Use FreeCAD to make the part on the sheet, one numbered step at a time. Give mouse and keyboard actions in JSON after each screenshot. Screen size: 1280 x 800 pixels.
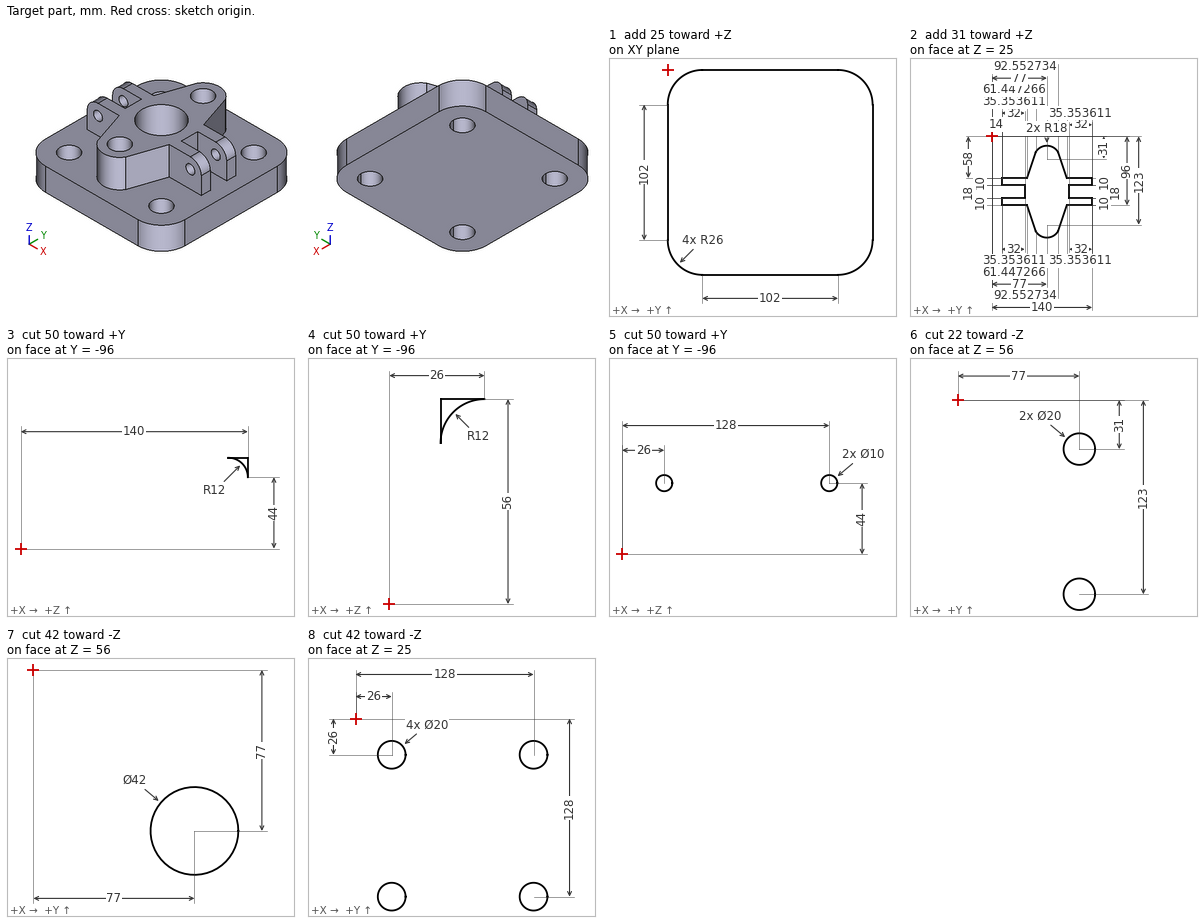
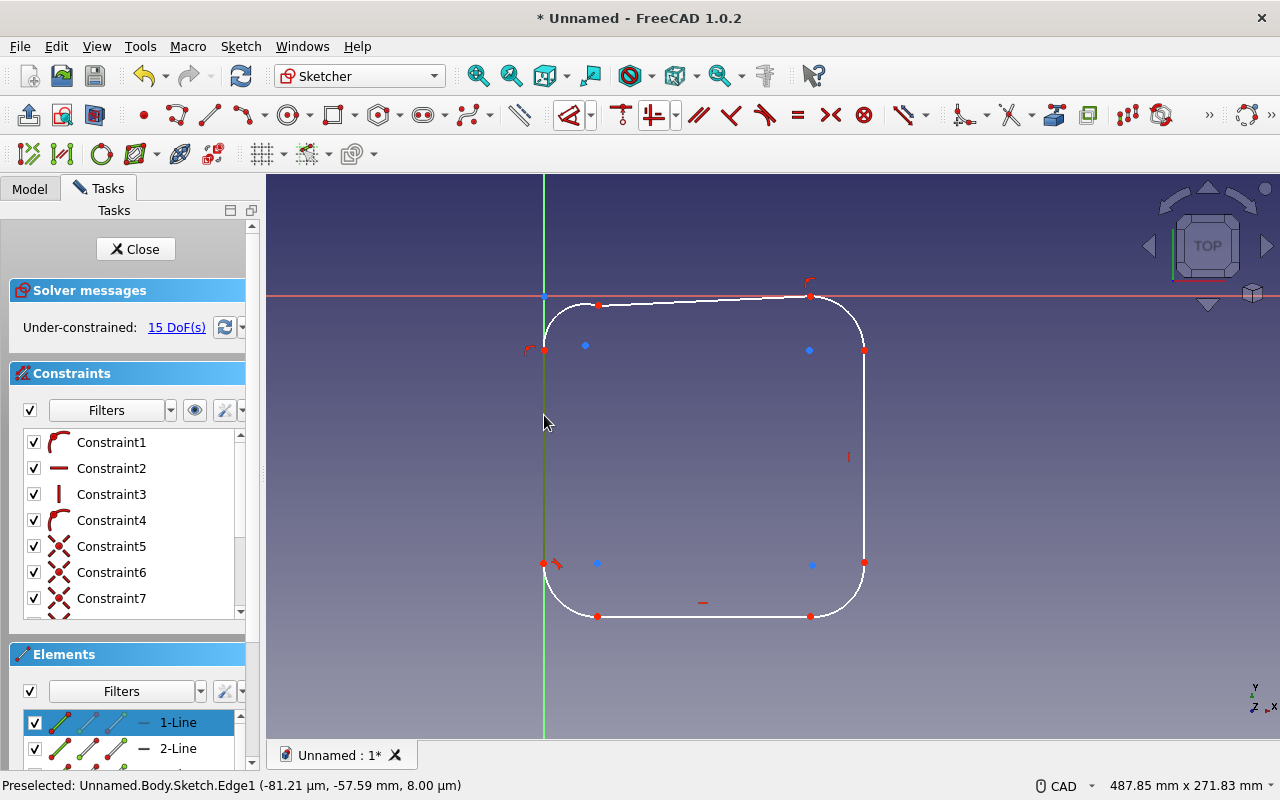
{"action": "scroll", "coordinate": [573, 306], "scroll_direction": "up", "scroll_amount": 2}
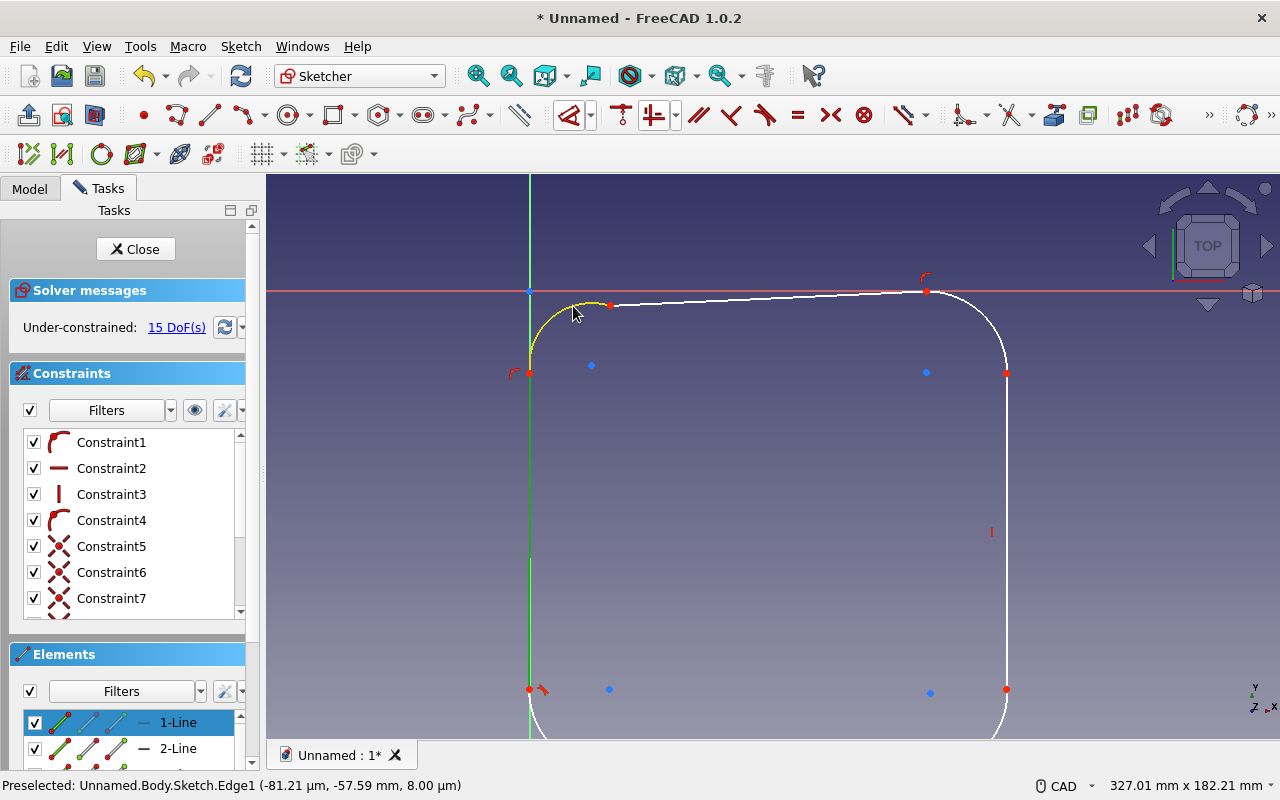
{"action": "left_click", "coordinate": [573, 306]}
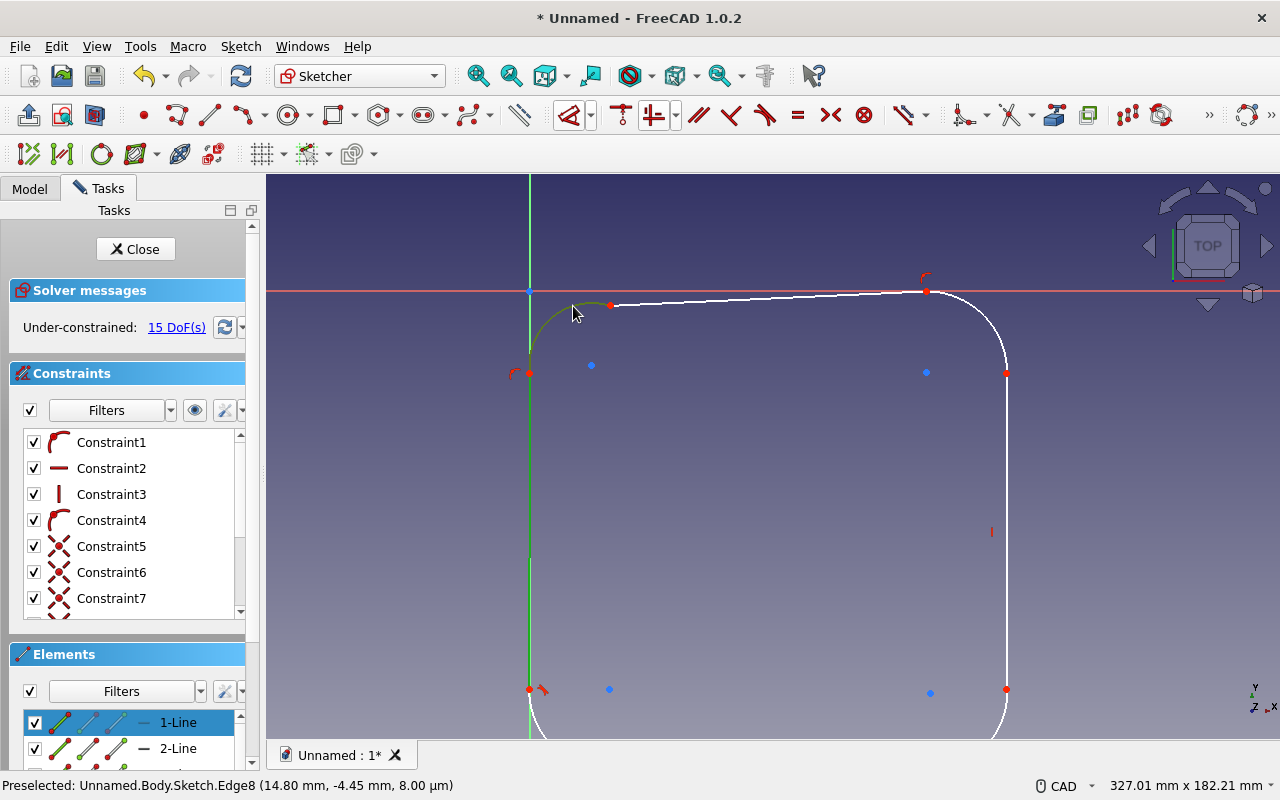
{"action": "left_click", "coordinate": [765, 116]}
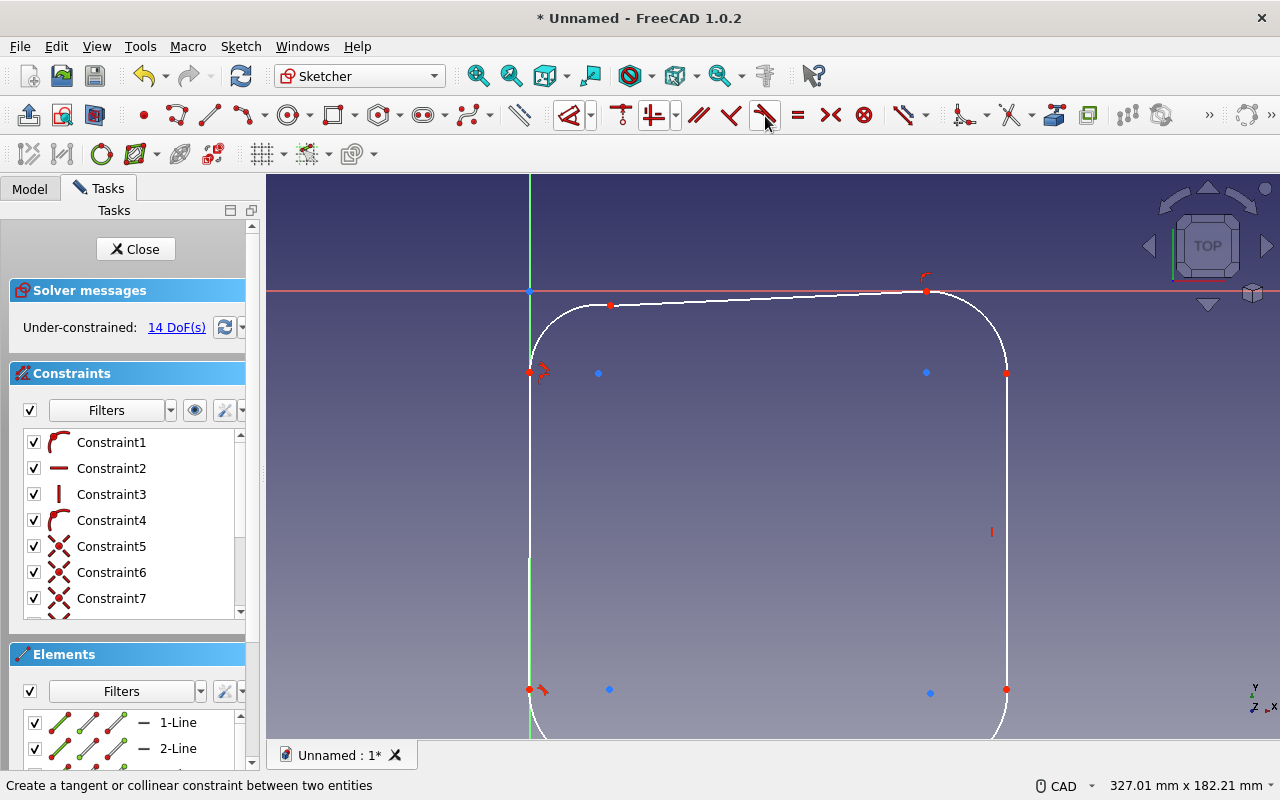
{"action": "scroll", "coordinate": [414, 202], "scroll_direction": "down", "scroll_amount": 1}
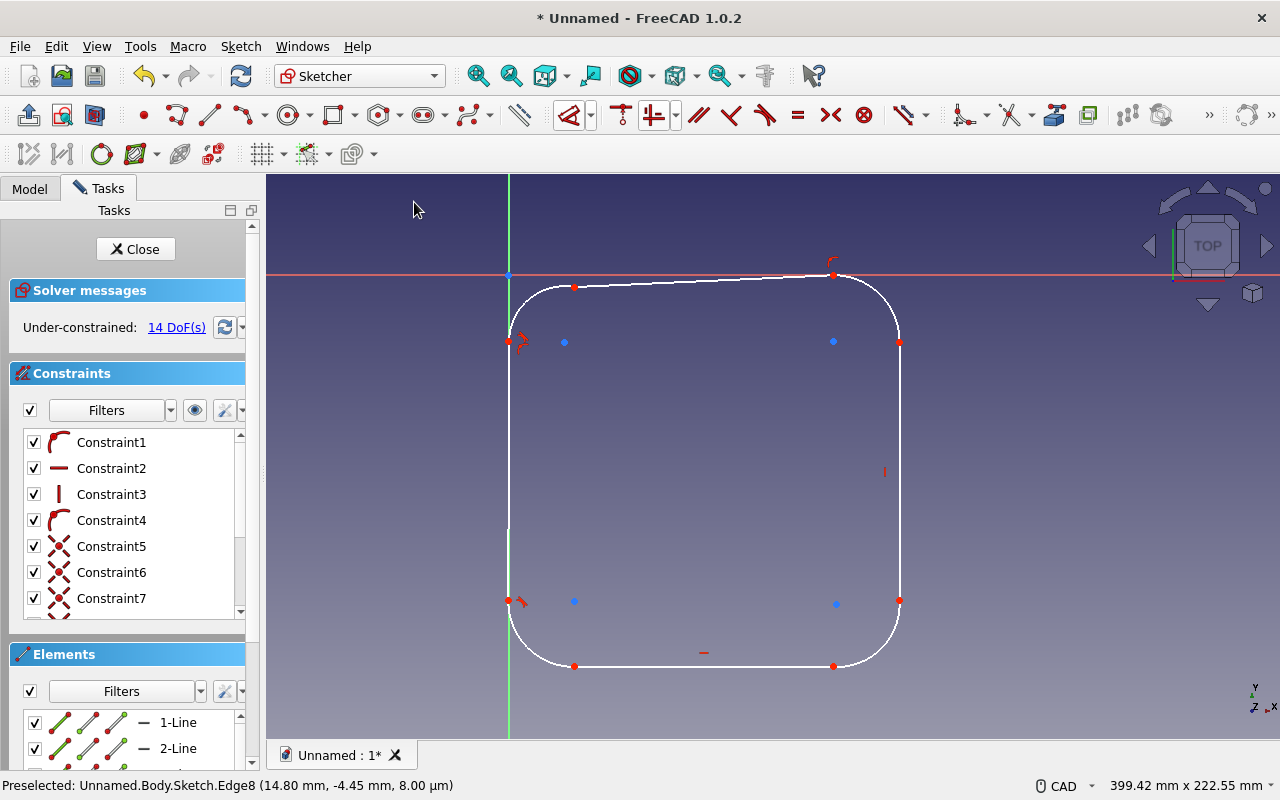
{"action": "left_click", "coordinate": [652, 667]}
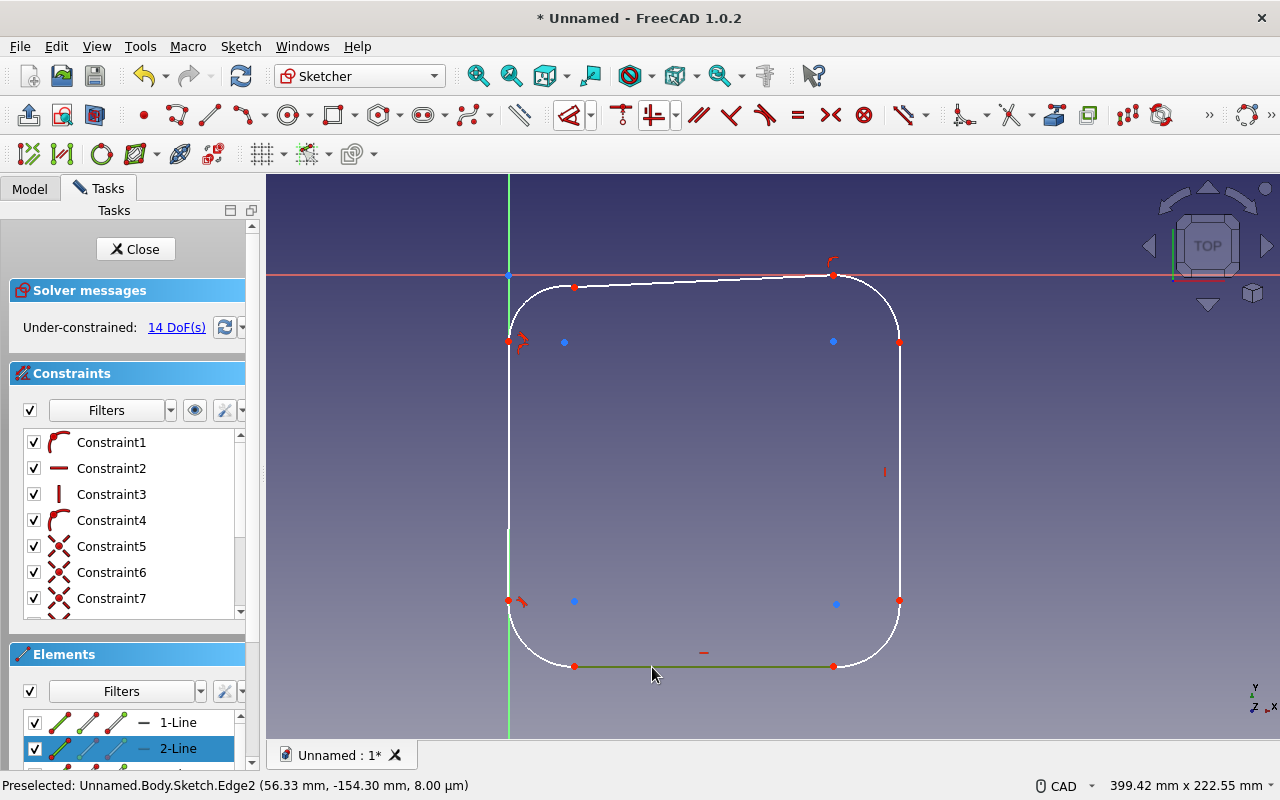
{"action": "left_click", "coordinate": [545, 660]}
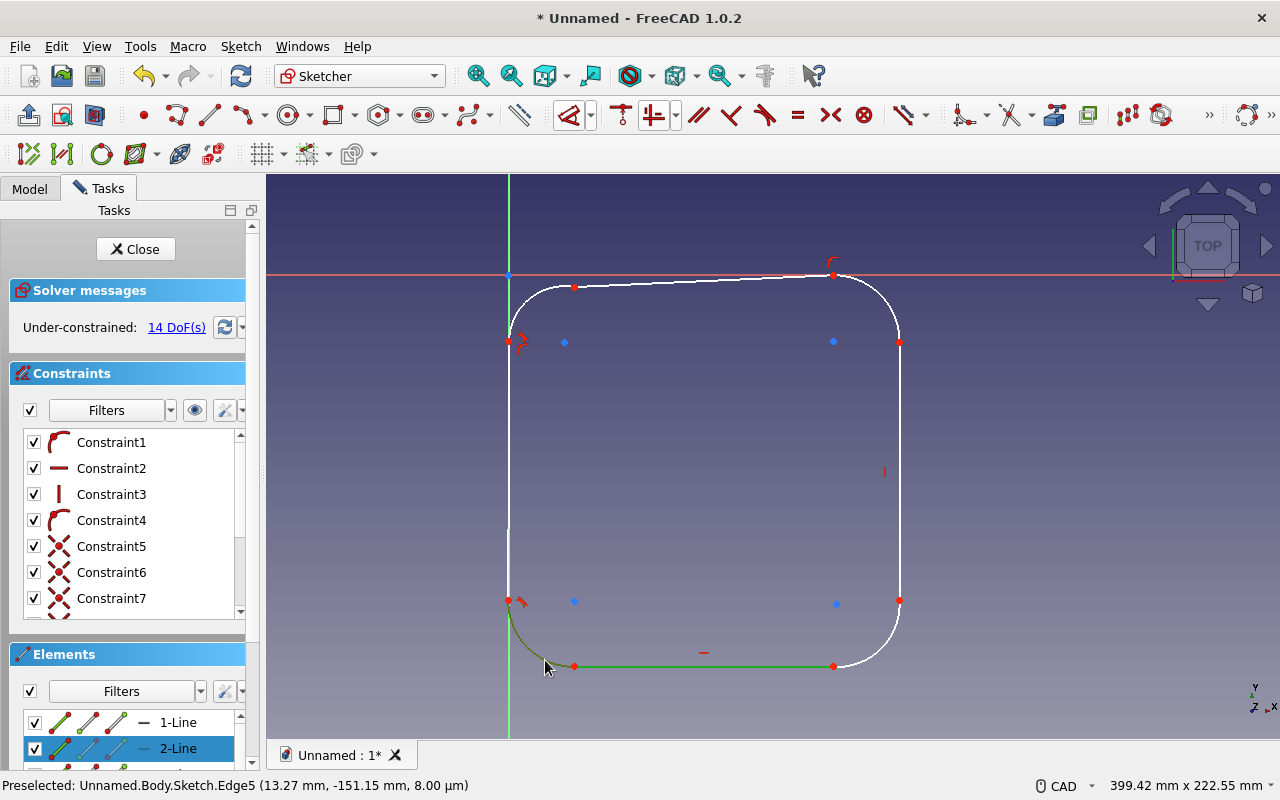
{"action": "left_click", "coordinate": [765, 116]}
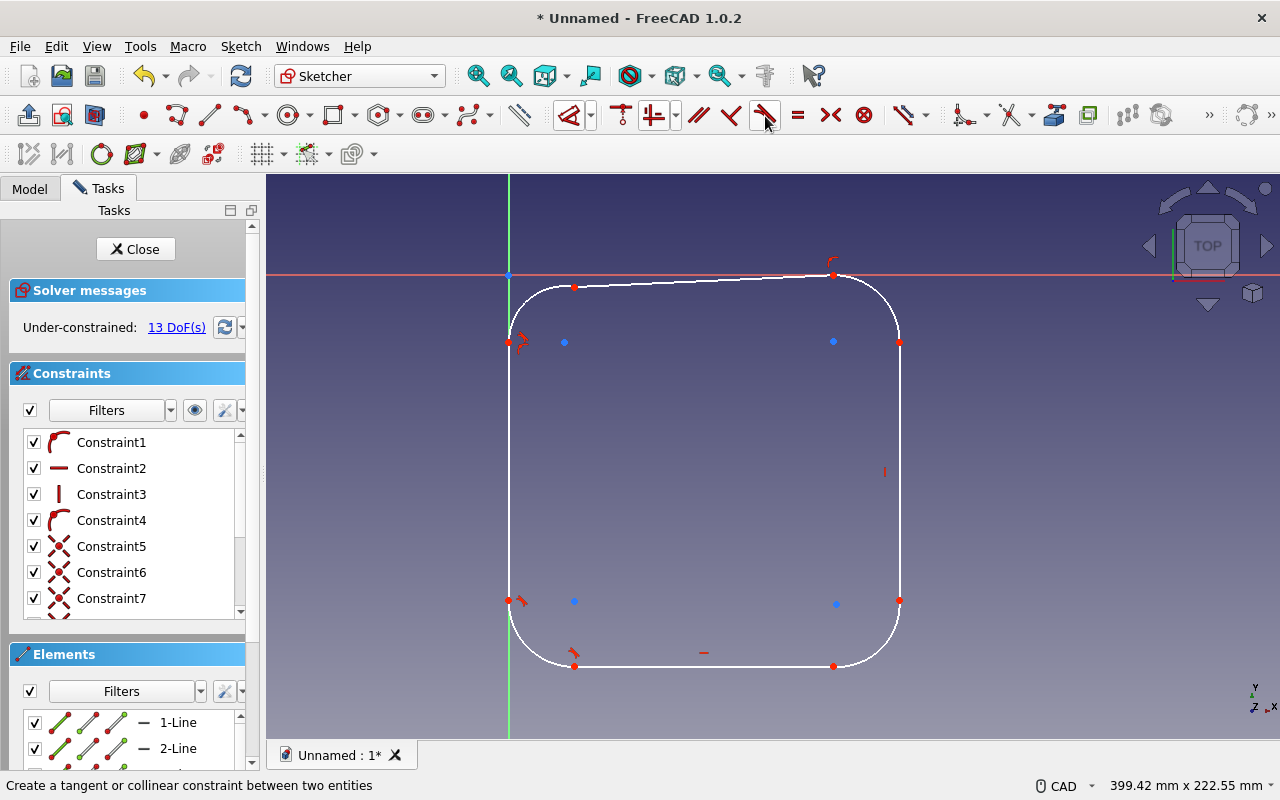
{"action": "left_click", "coordinate": [652, 667]}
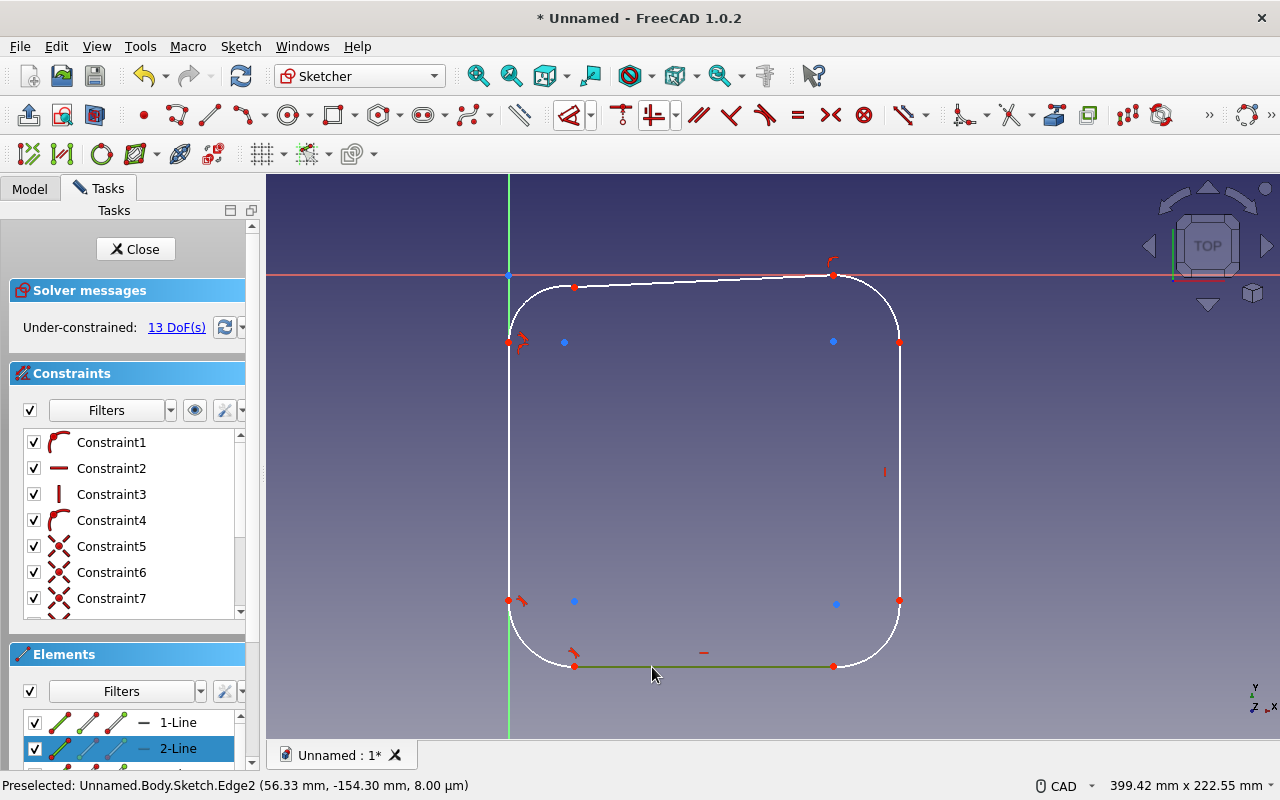
{"action": "left_click", "coordinate": [864, 661]}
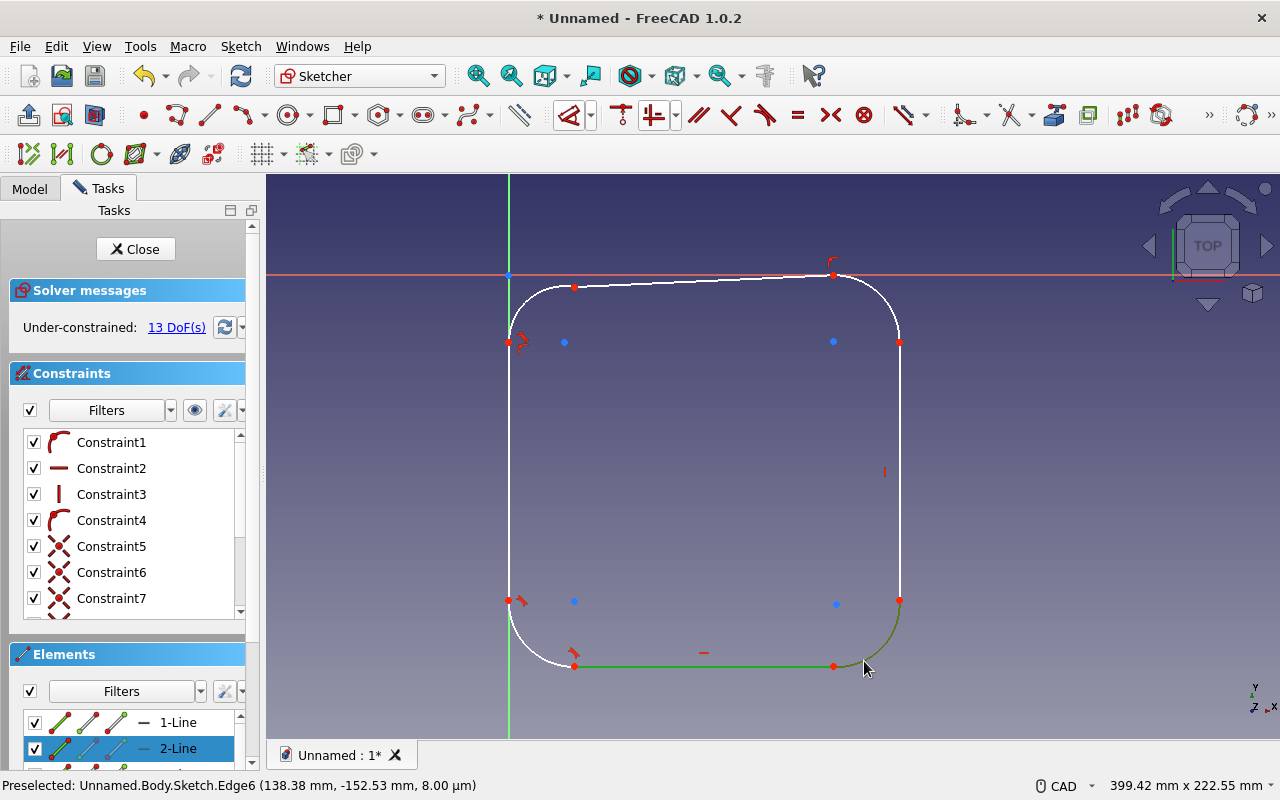
{"action": "left_click", "coordinate": [765, 116]}